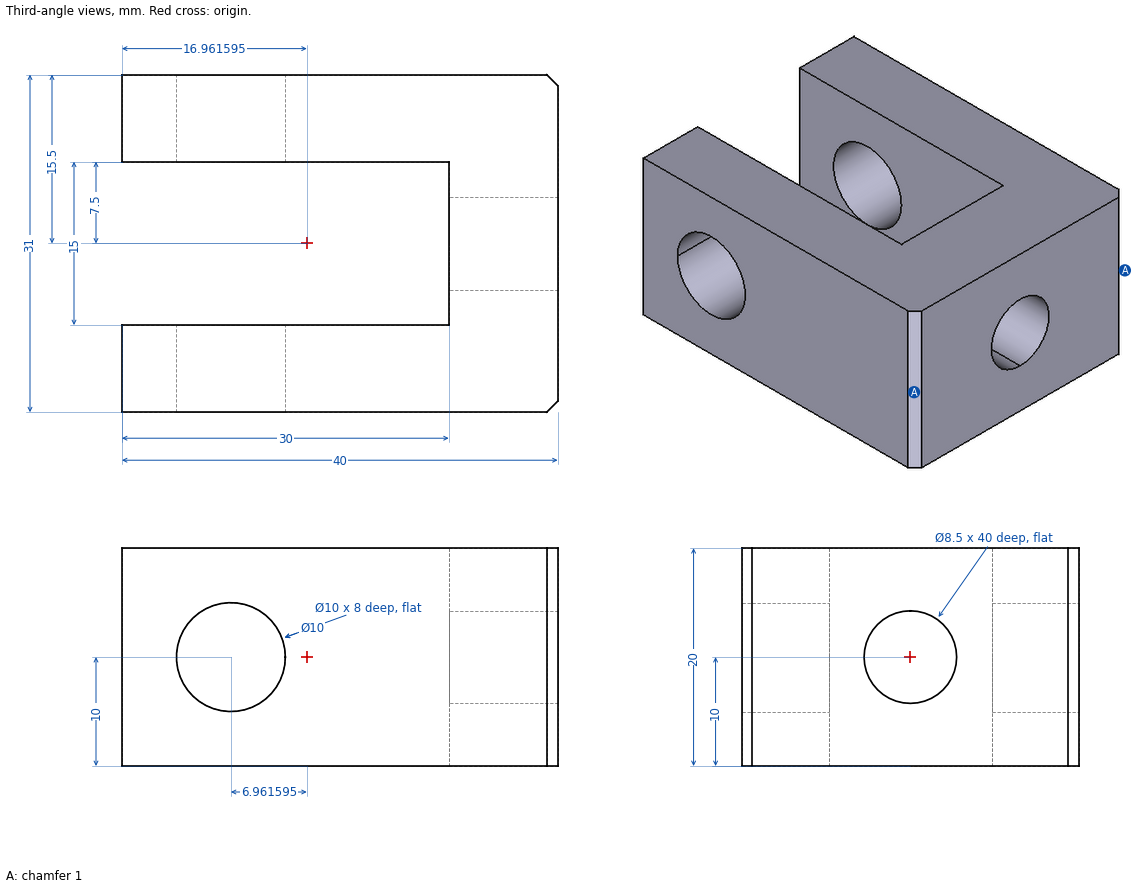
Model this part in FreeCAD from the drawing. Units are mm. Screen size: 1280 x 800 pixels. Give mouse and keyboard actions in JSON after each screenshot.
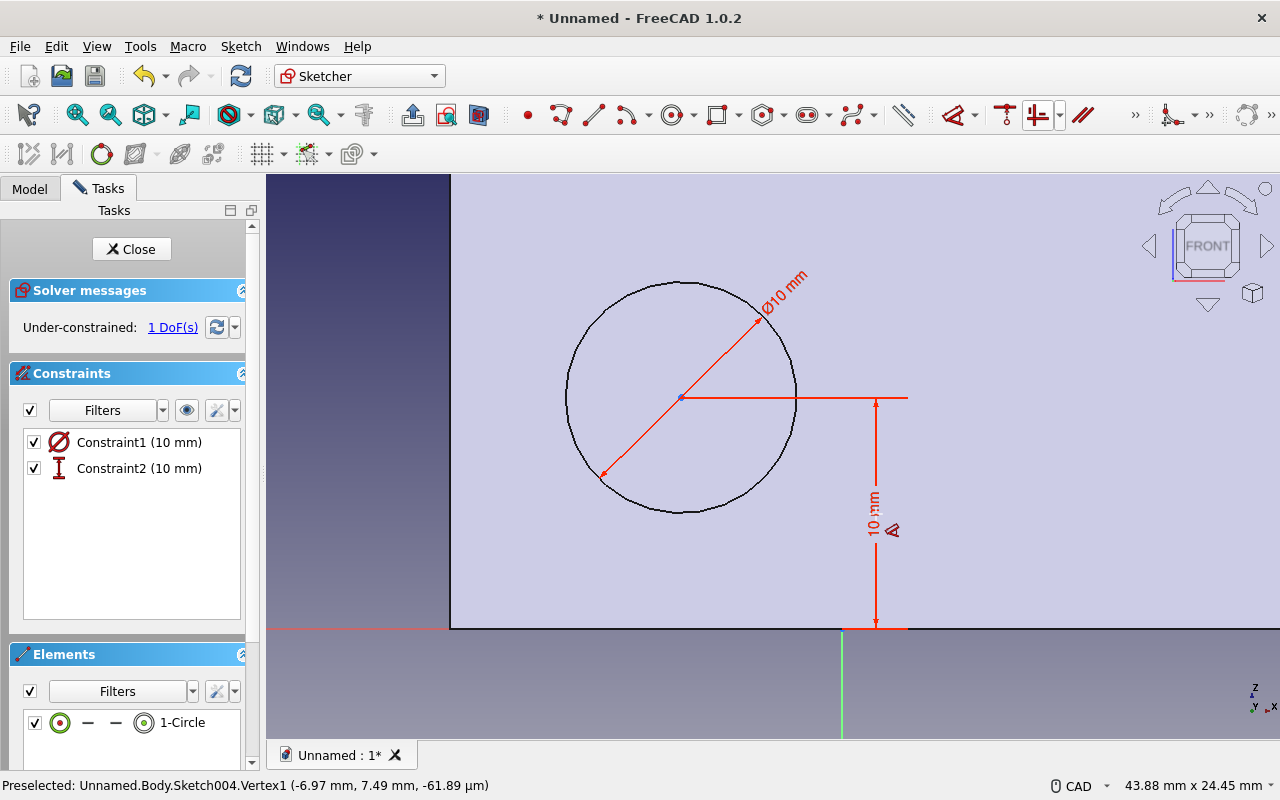
{"action": "left_click", "coordinate": [681, 398]}
{"action": "left_click", "coordinate": [762, 663]}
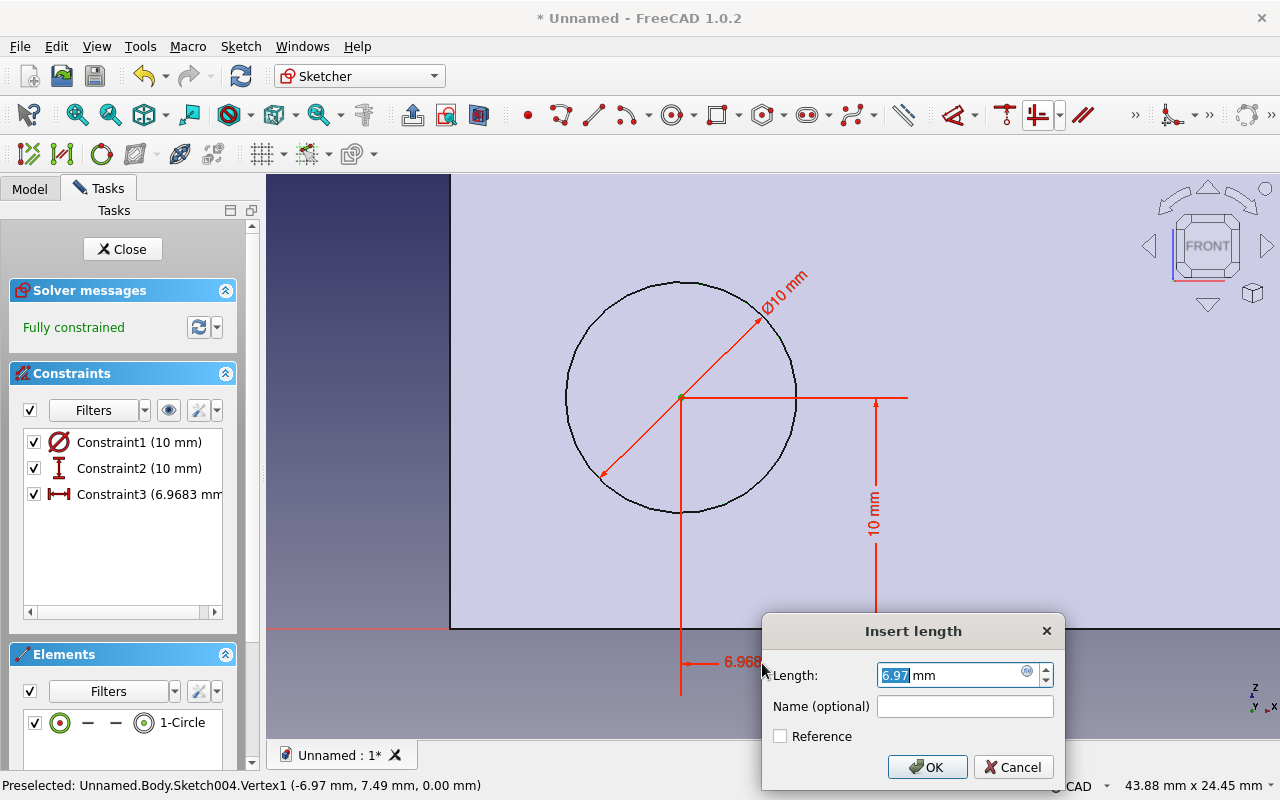
{"action": "type", "text": "6.961595"}
{"action": "key", "text": "Return"}
{"action": "key", "text": "Escape"}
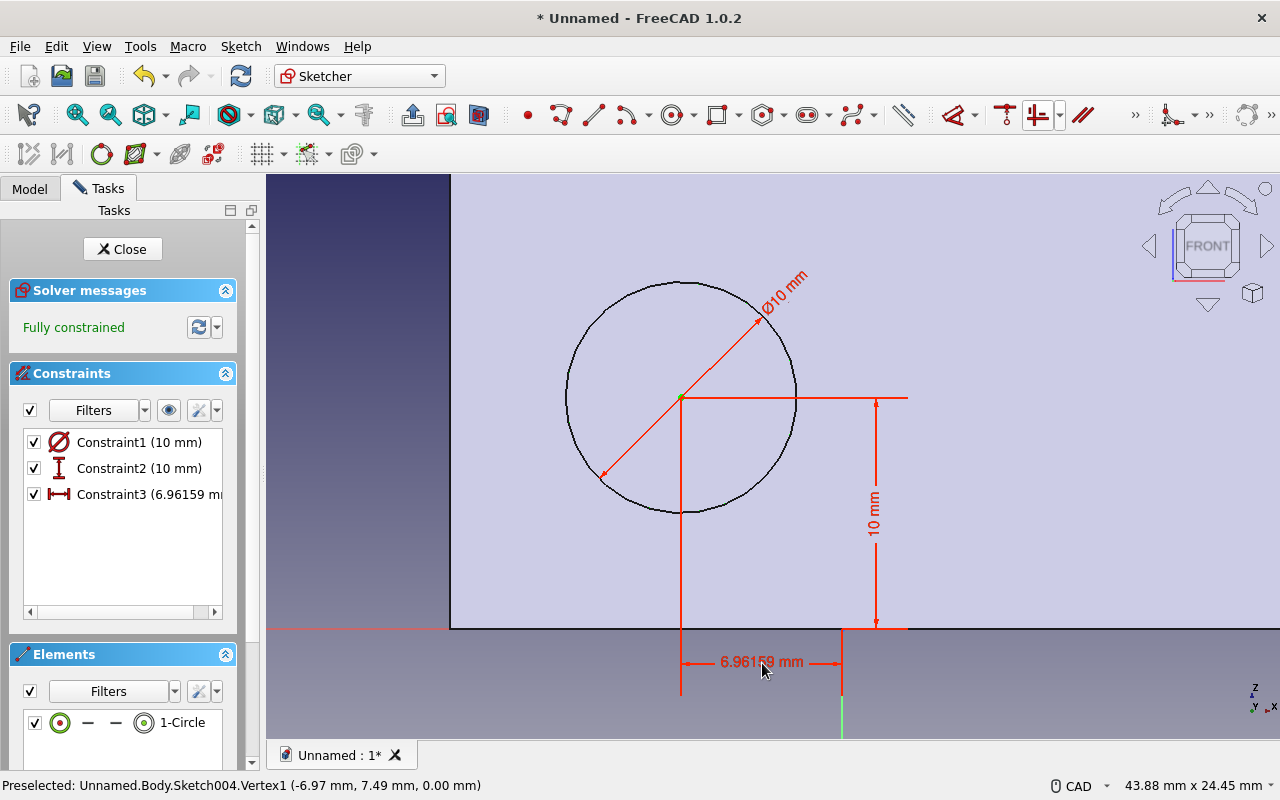
{"action": "left_click", "coordinate": [123, 249]}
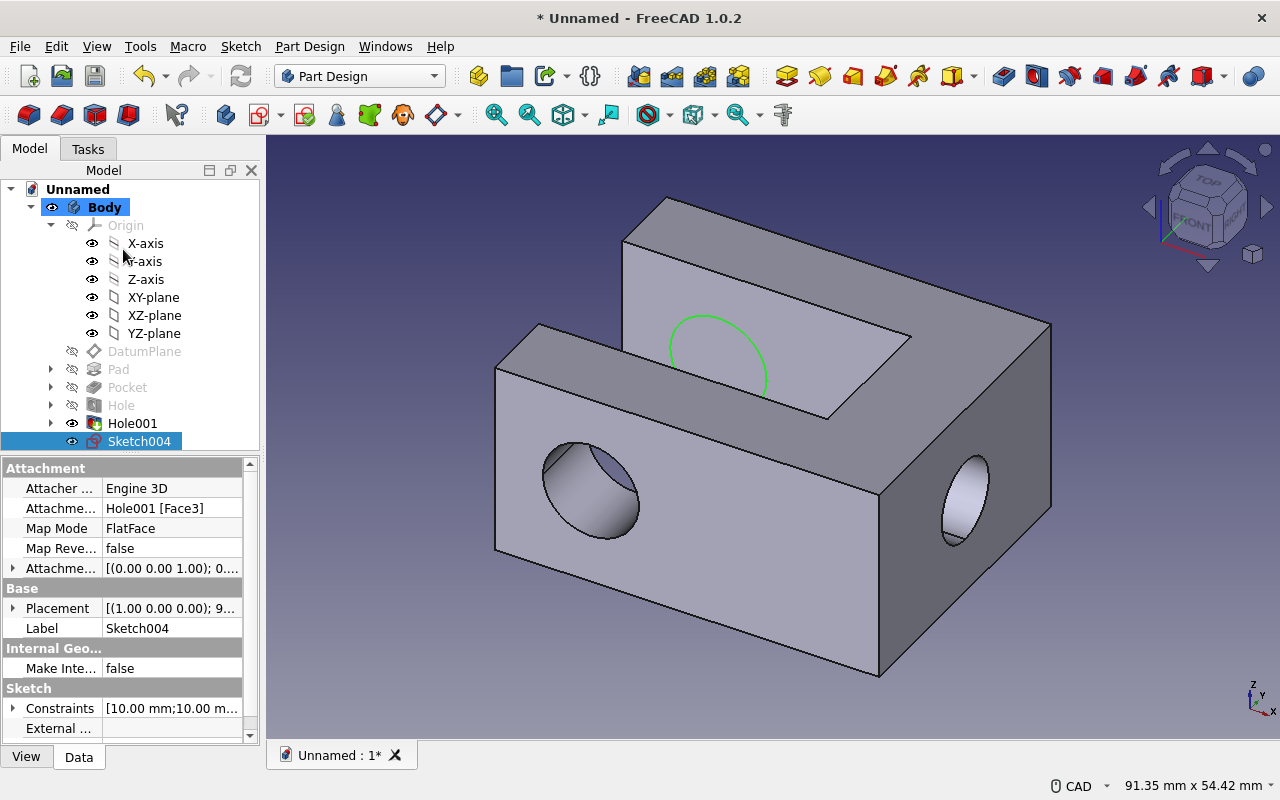
{"action": "left_click", "coordinate": [1004, 76]}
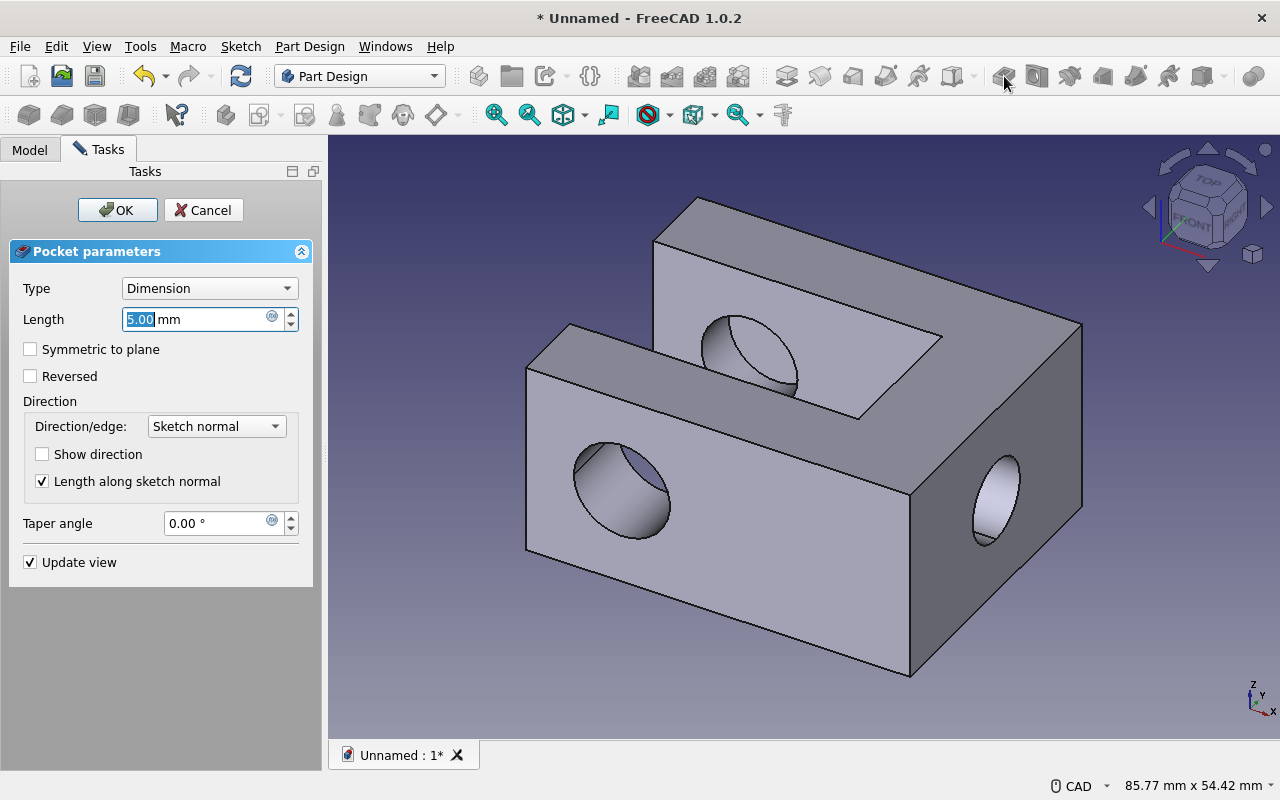
{"action": "left_click", "coordinate": [210, 288]}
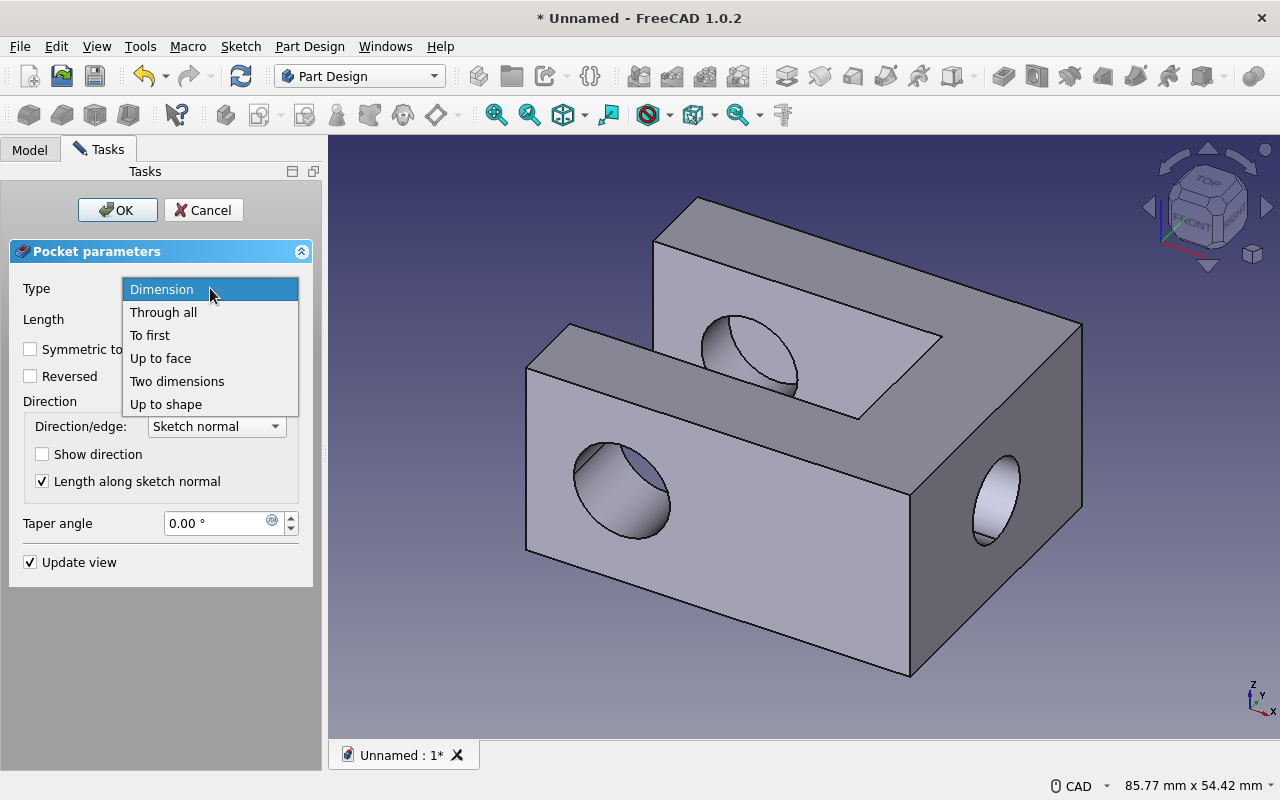
{"action": "left_click", "coordinate": [208, 312]}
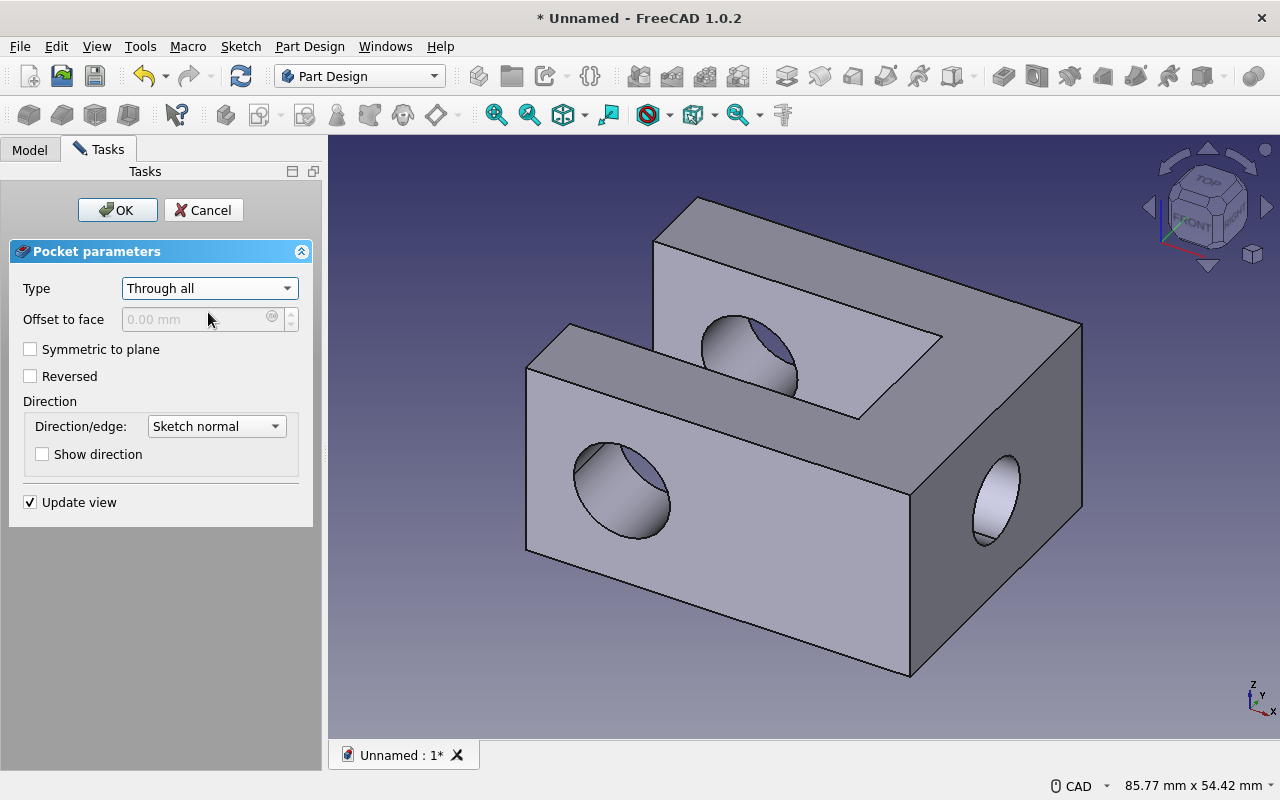
{"action": "left_click", "coordinate": [118, 210]}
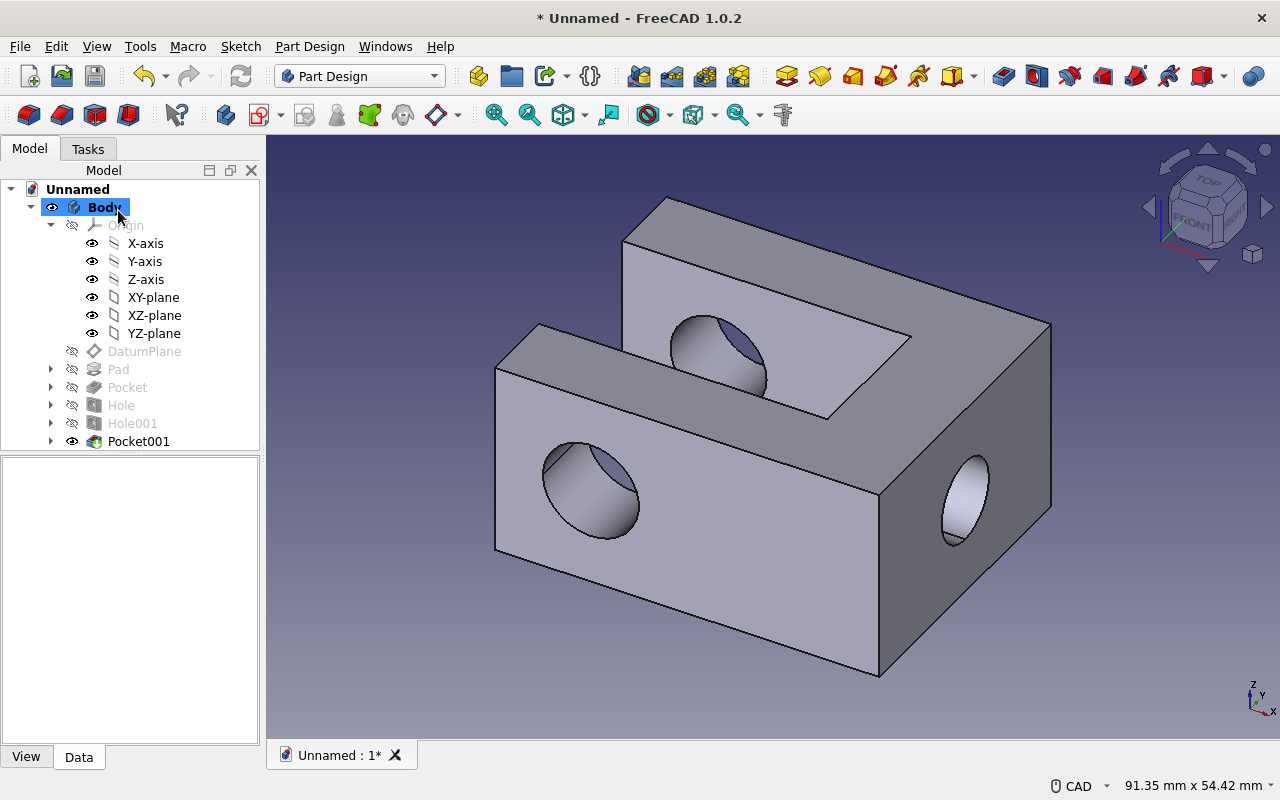
{"action": "left_click", "coordinate": [879, 585]}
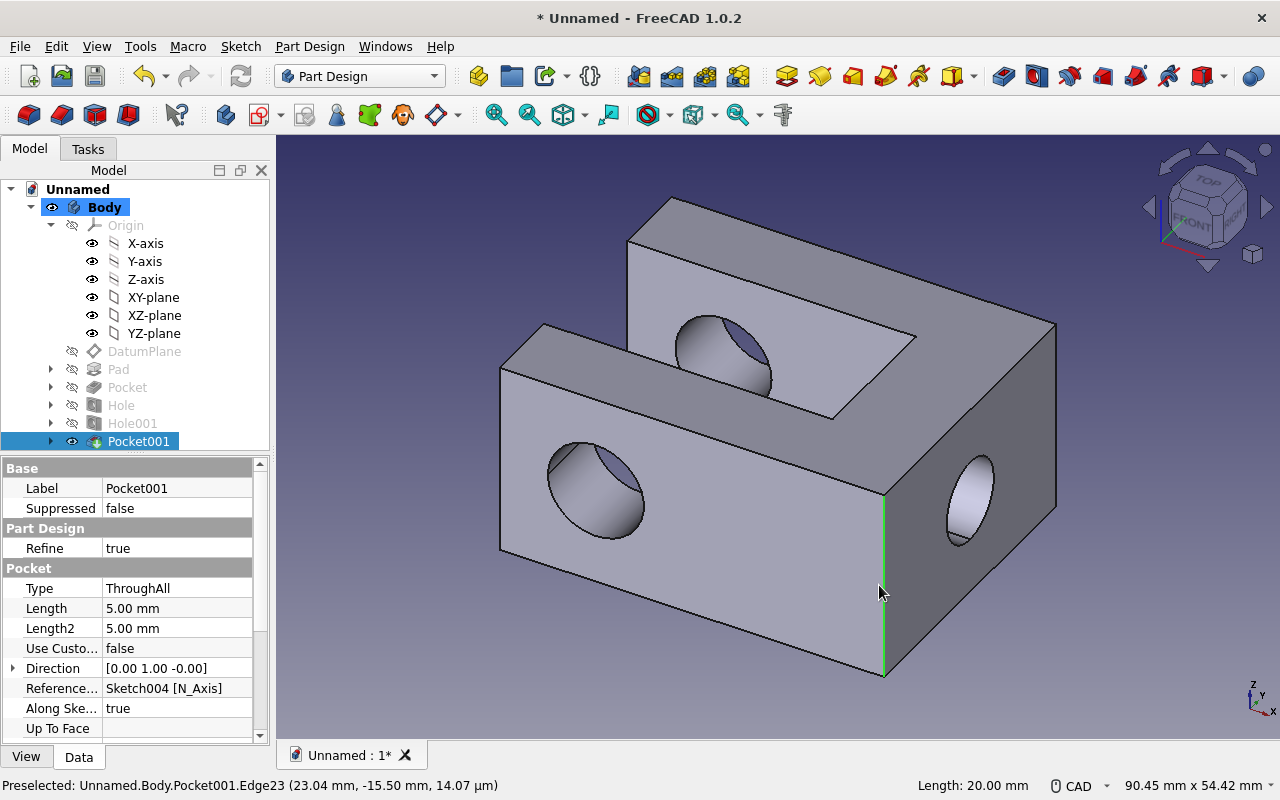
{"action": "key", "text": "0"}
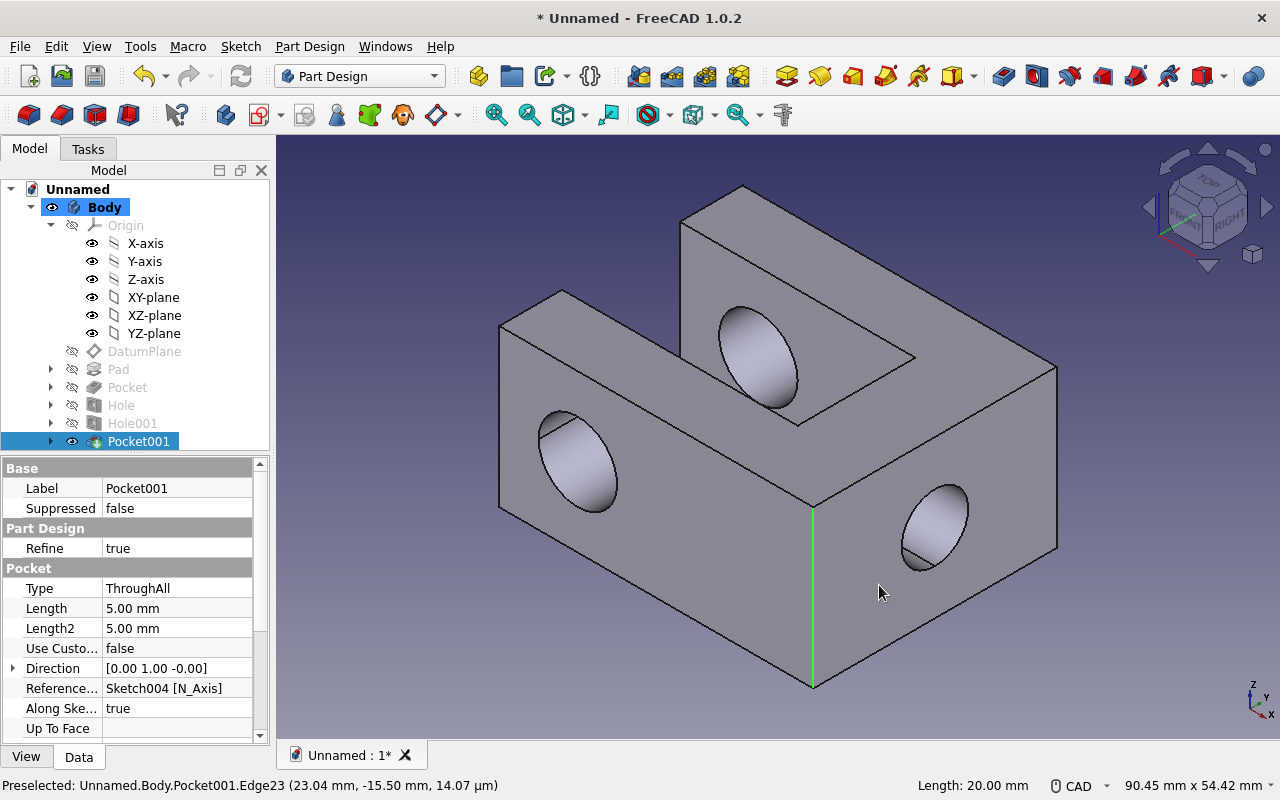
{"action": "key", "text": "2"}